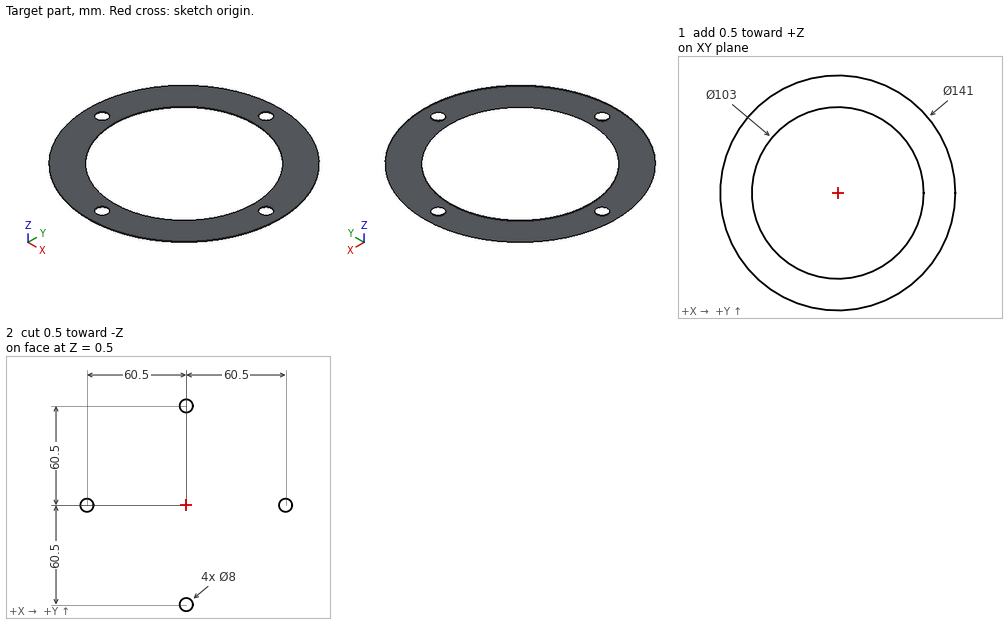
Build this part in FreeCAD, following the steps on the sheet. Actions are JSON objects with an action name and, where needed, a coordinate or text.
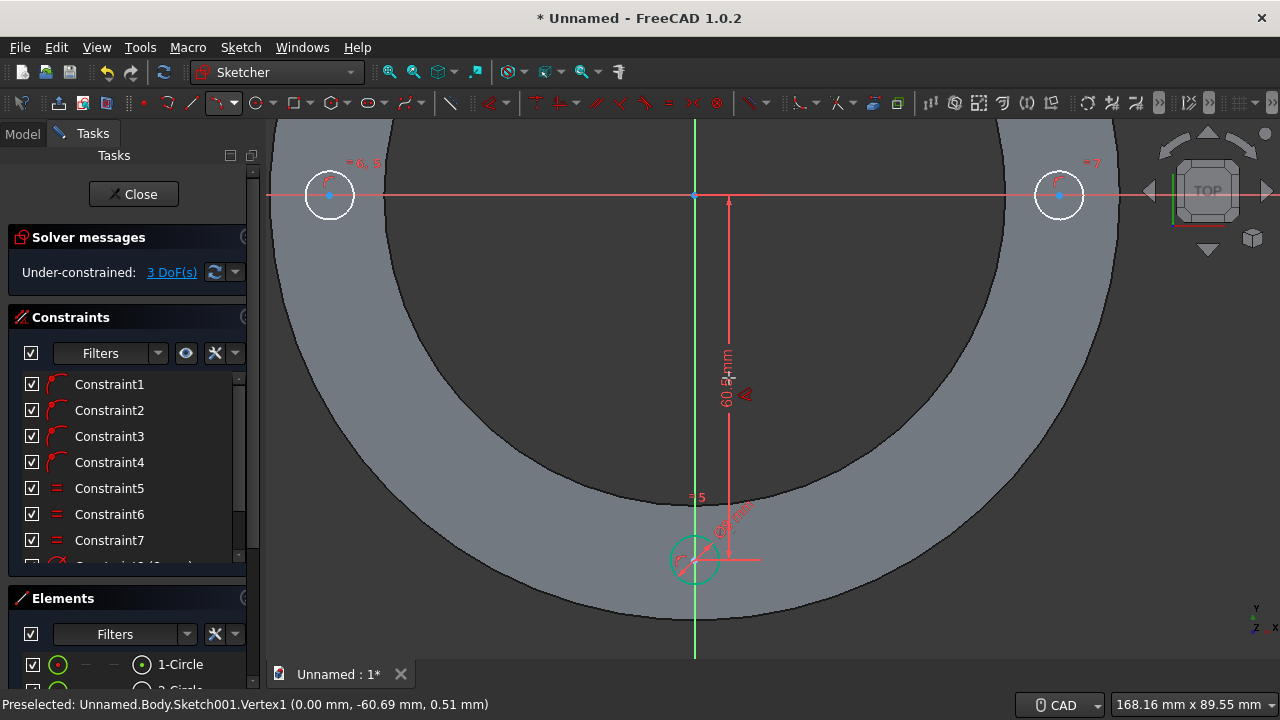
{"action": "left_click", "coordinate": [330, 195]}
{"action": "left_click", "coordinate": [512, 229]}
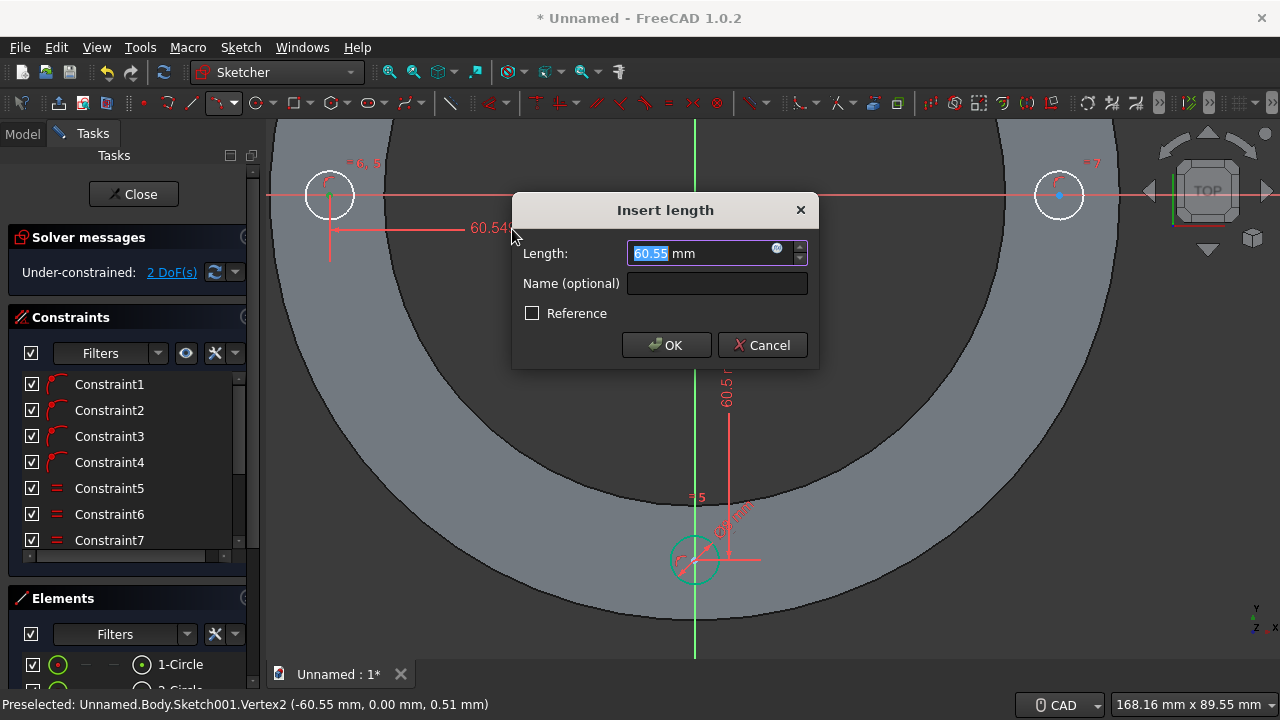
{"action": "type", "text": "60.5"}
{"action": "key", "text": "Return"}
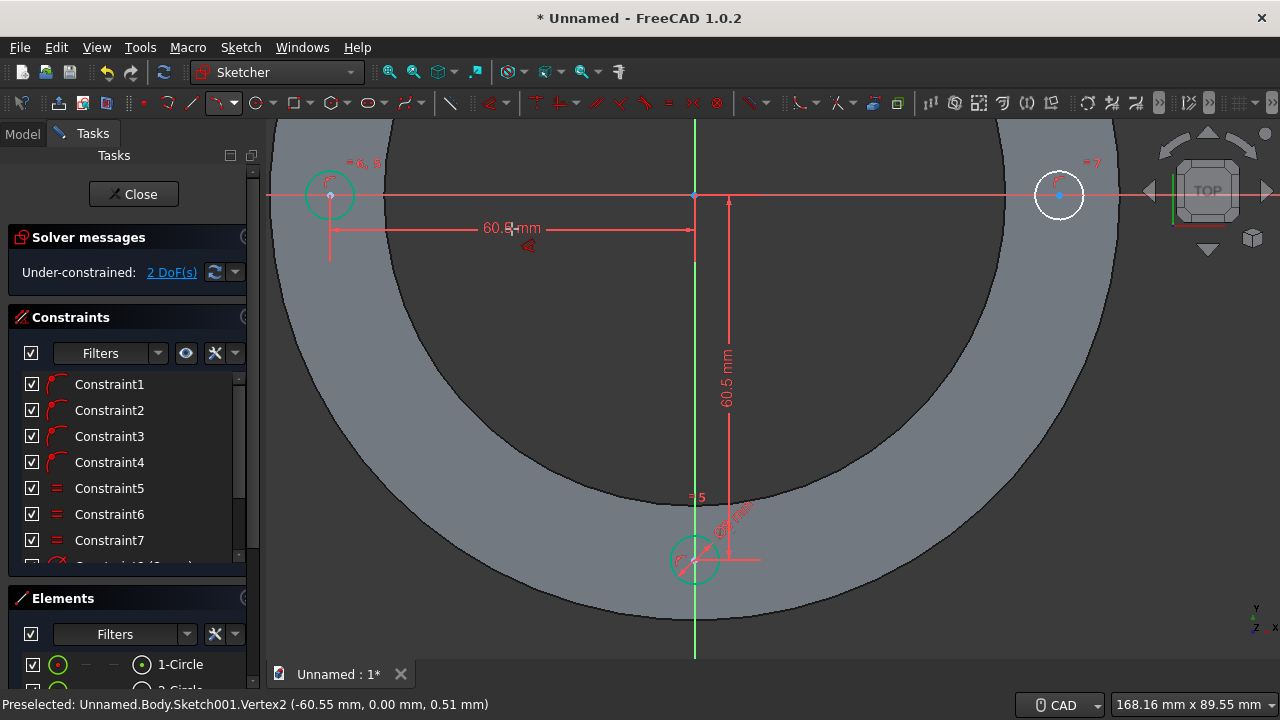
{"action": "scroll", "coordinate": [712, 547], "scroll_direction": "down", "scroll_amount": 4}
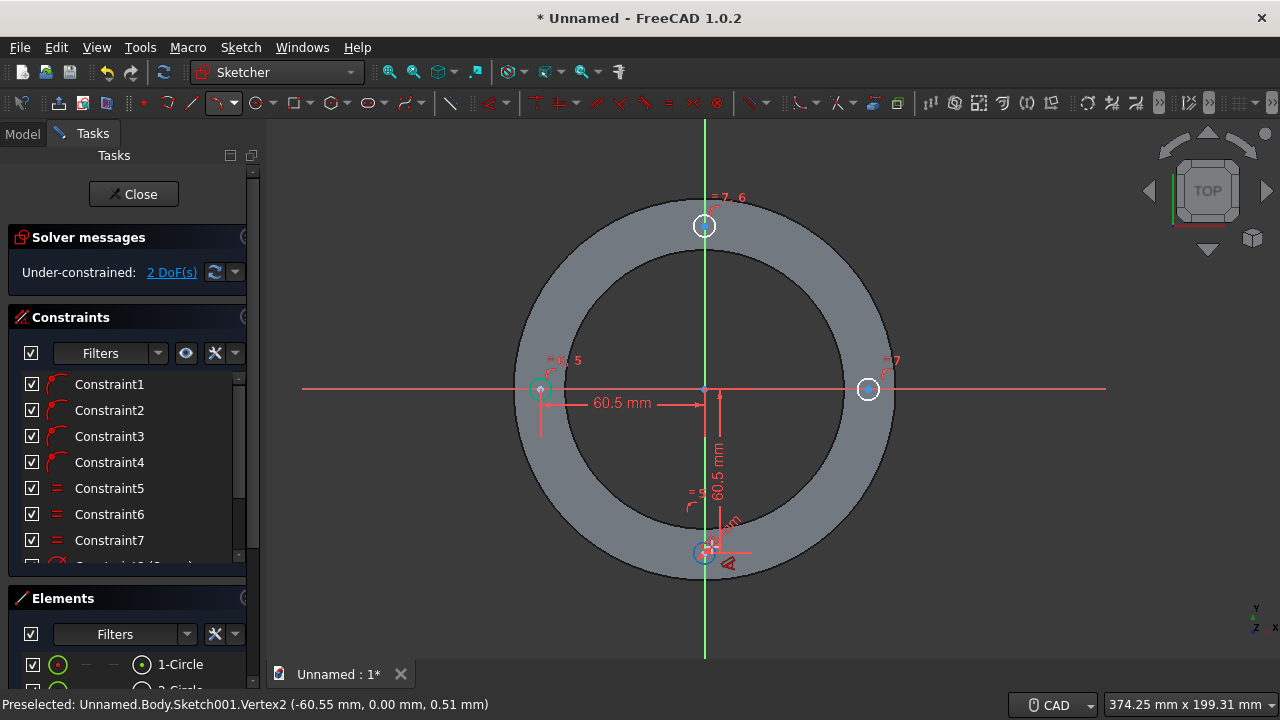
{"action": "left_click", "coordinate": [705, 226]}
{"action": "left_click", "coordinate": [739, 308]}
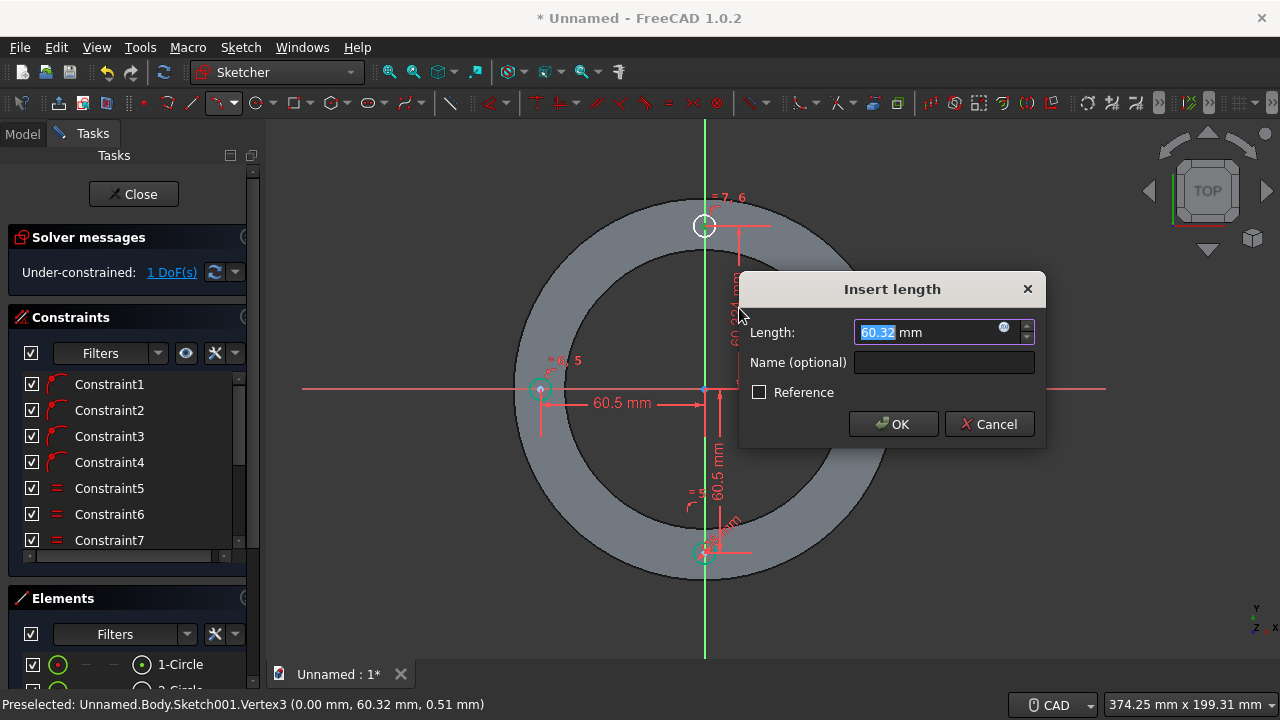
{"action": "type", "text": "60.5"}
{"action": "key", "text": "Return"}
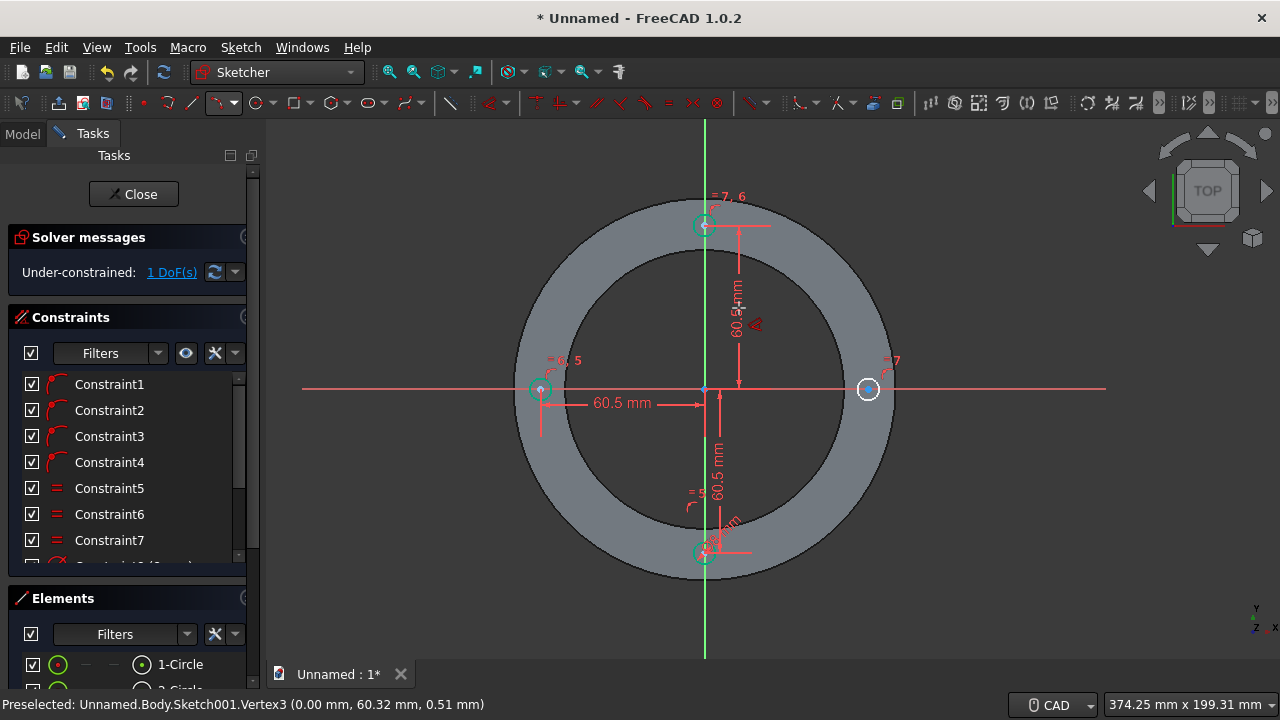
{"action": "left_click", "coordinate": [868, 389]}
{"action": "left_click", "coordinate": [786, 423]}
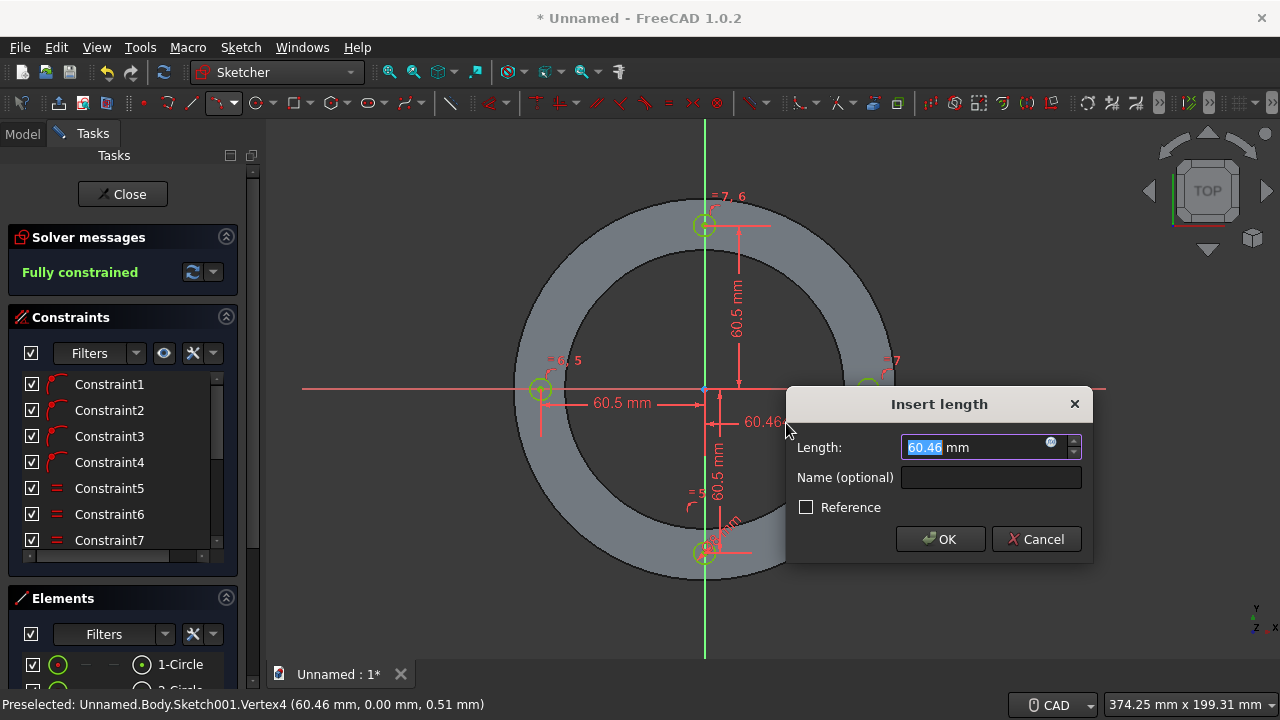
{"action": "type", "text": "60.5"}
{"action": "key", "text": "Return"}
{"action": "key", "text": "Escape"}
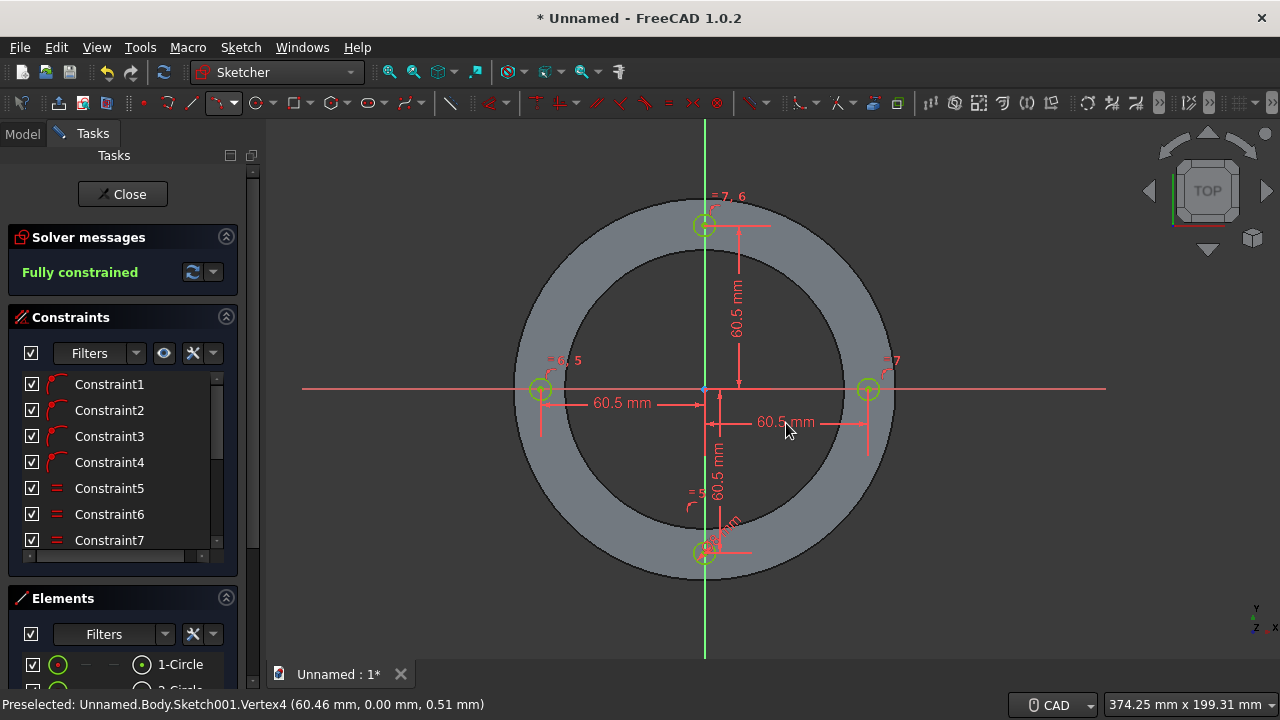
{"action": "left_click", "coordinate": [123, 194]}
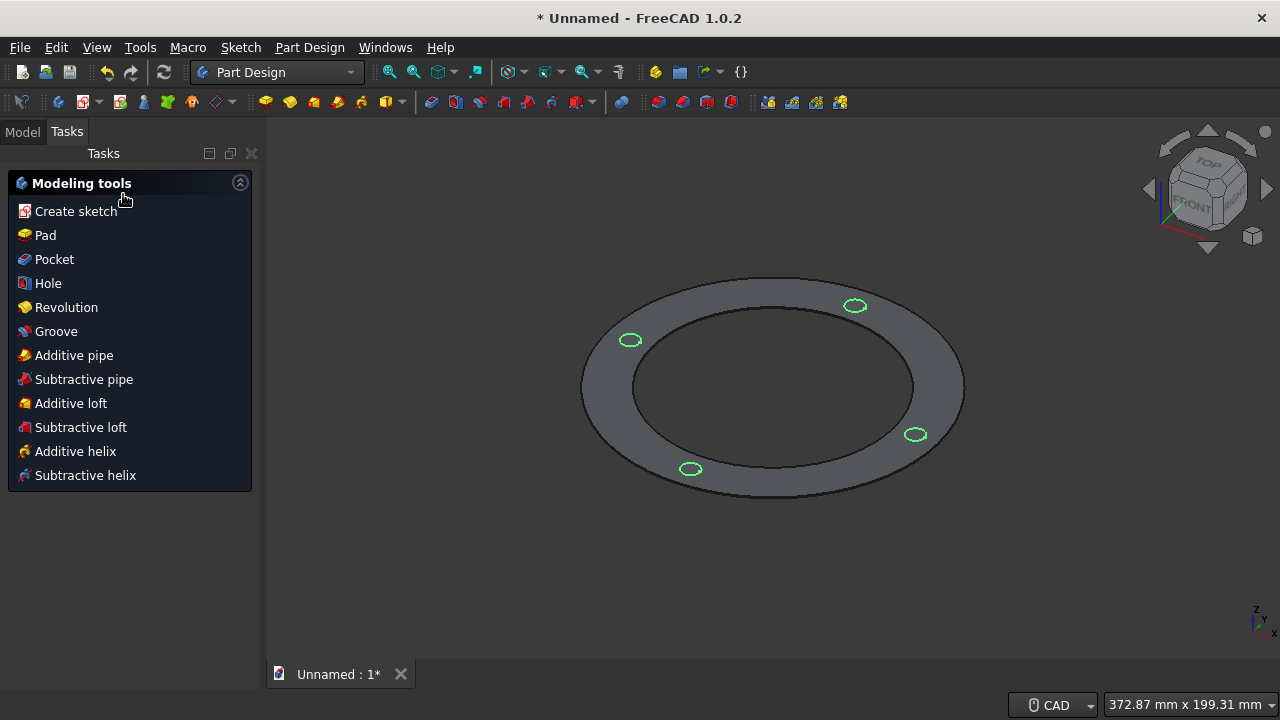
{"action": "left_click", "coordinate": [432, 102]}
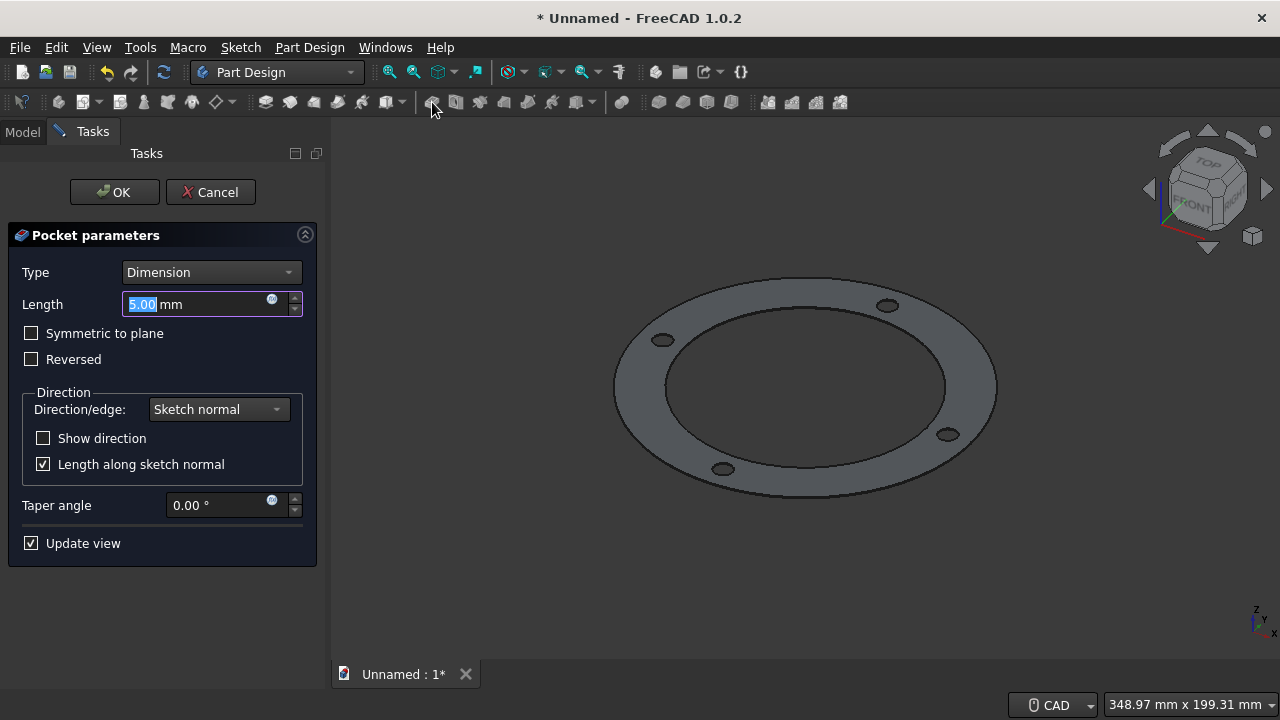
{"action": "type", "text": "0.5"}
{"action": "key", "text": "Tab"}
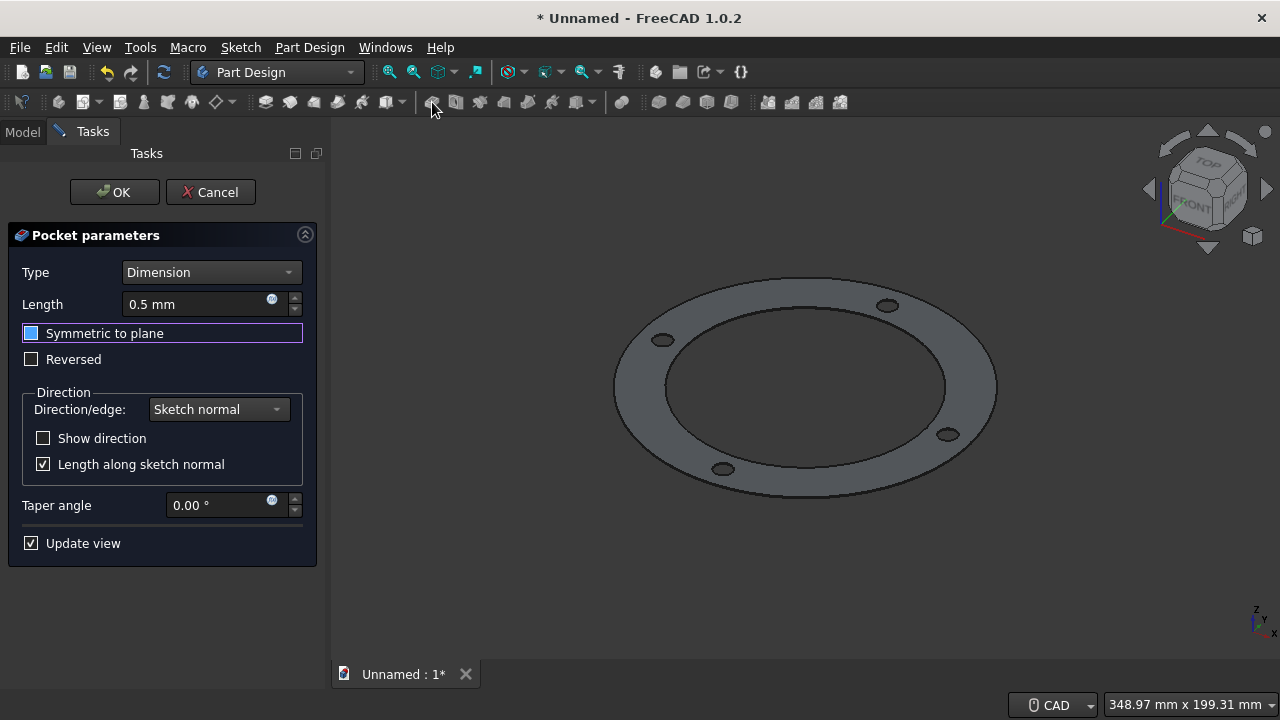
{"action": "left_click", "coordinate": [115, 192]}